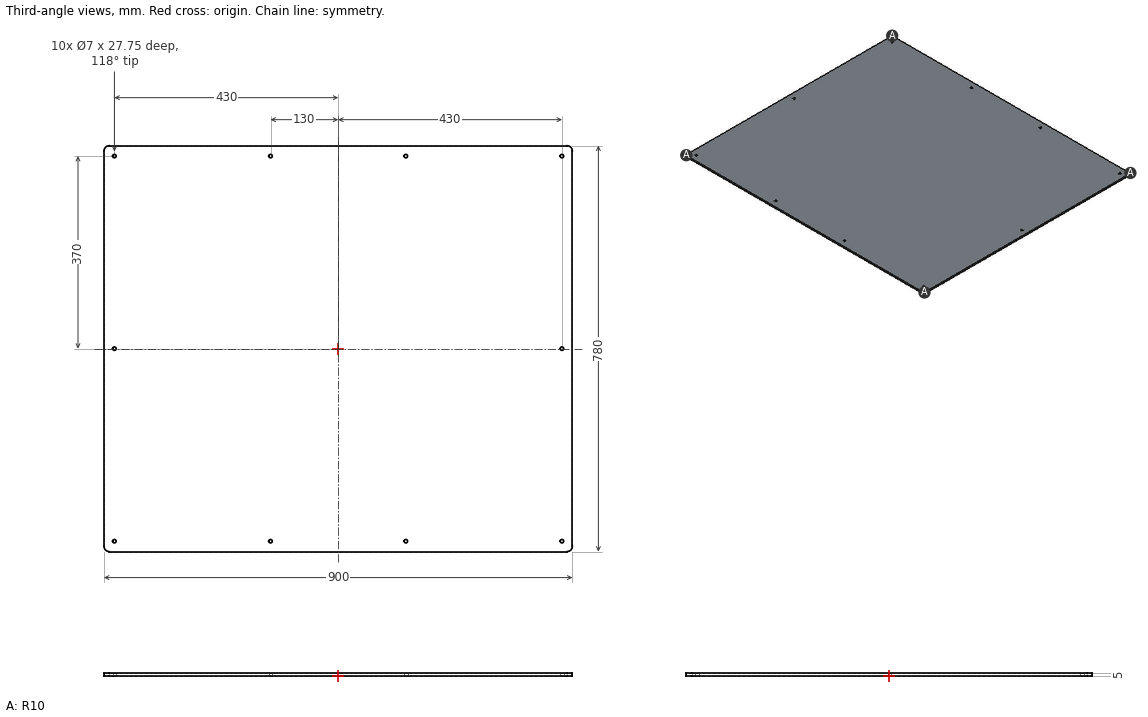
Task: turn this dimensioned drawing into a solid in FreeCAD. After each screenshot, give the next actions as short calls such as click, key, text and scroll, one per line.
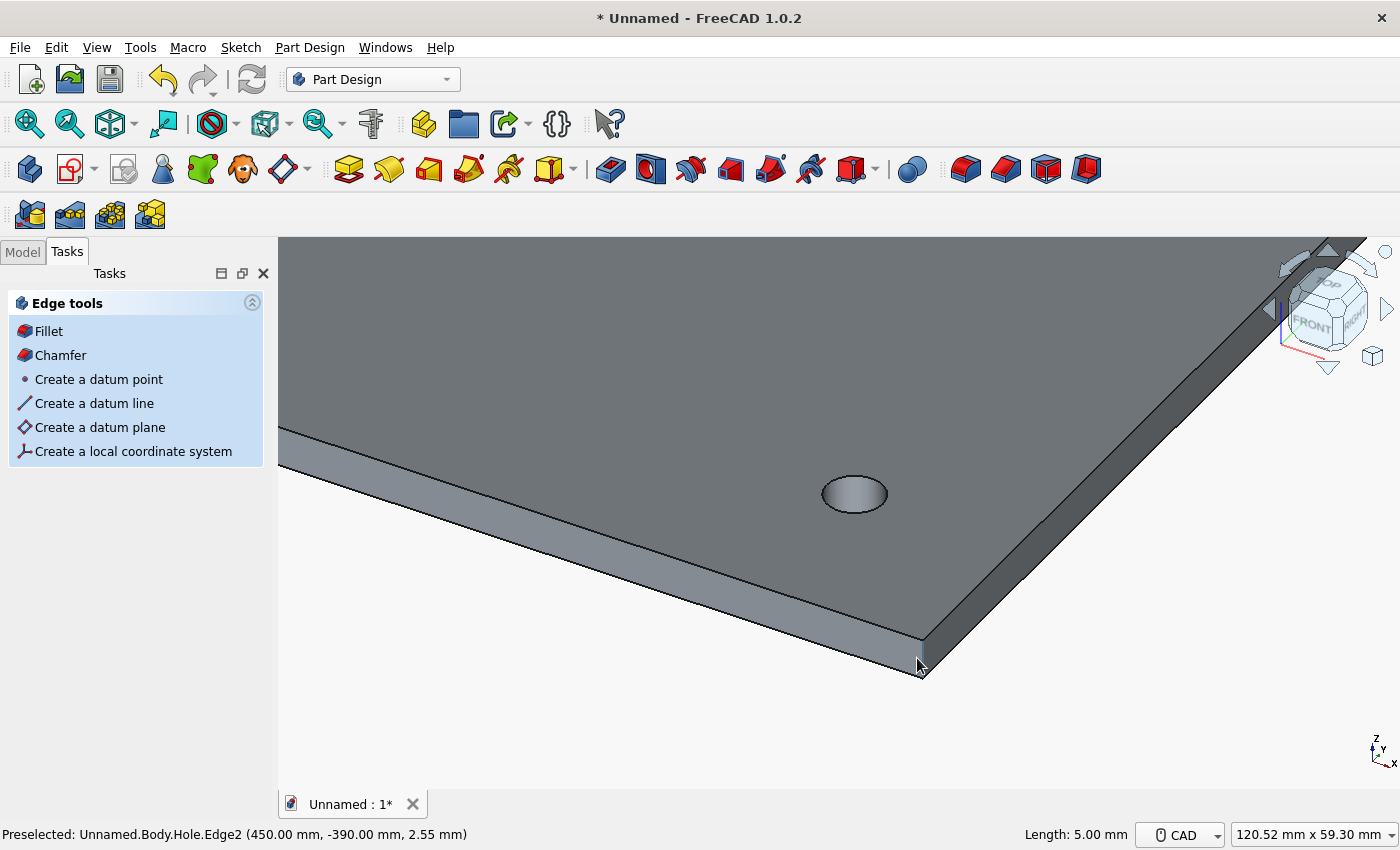
click(30, 124)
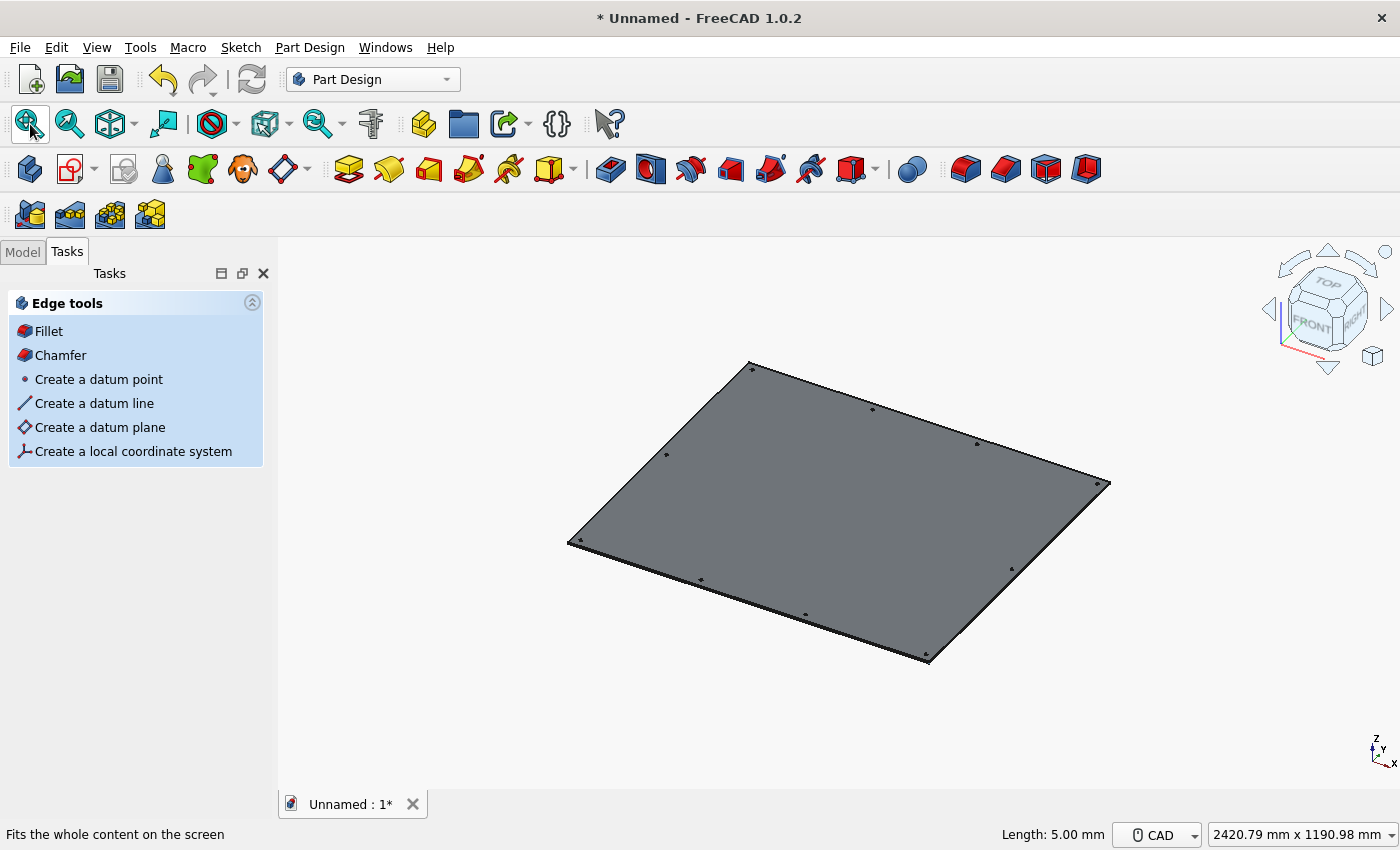
key(0)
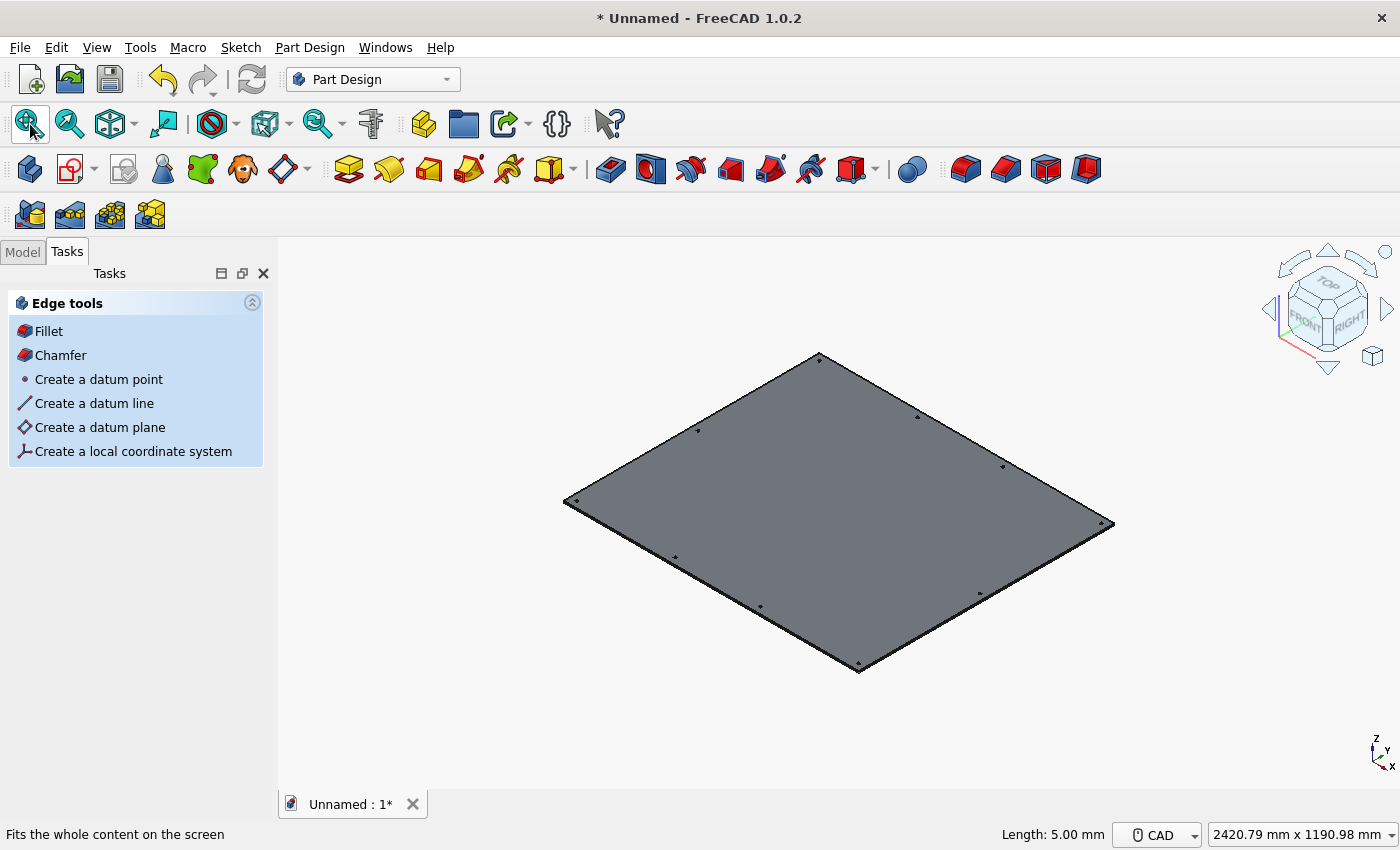
scroll(564, 501, up, 15)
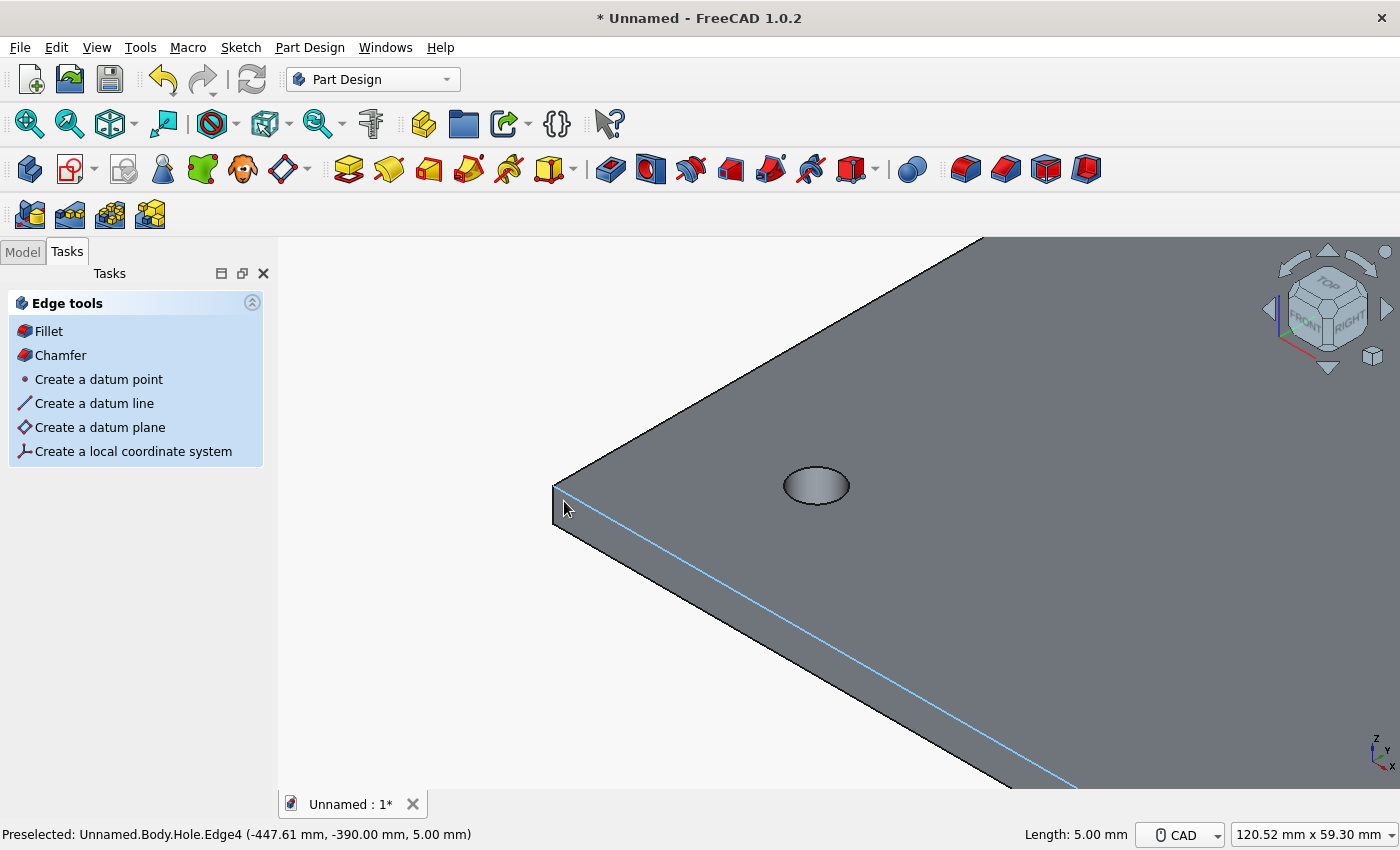
click(30, 124)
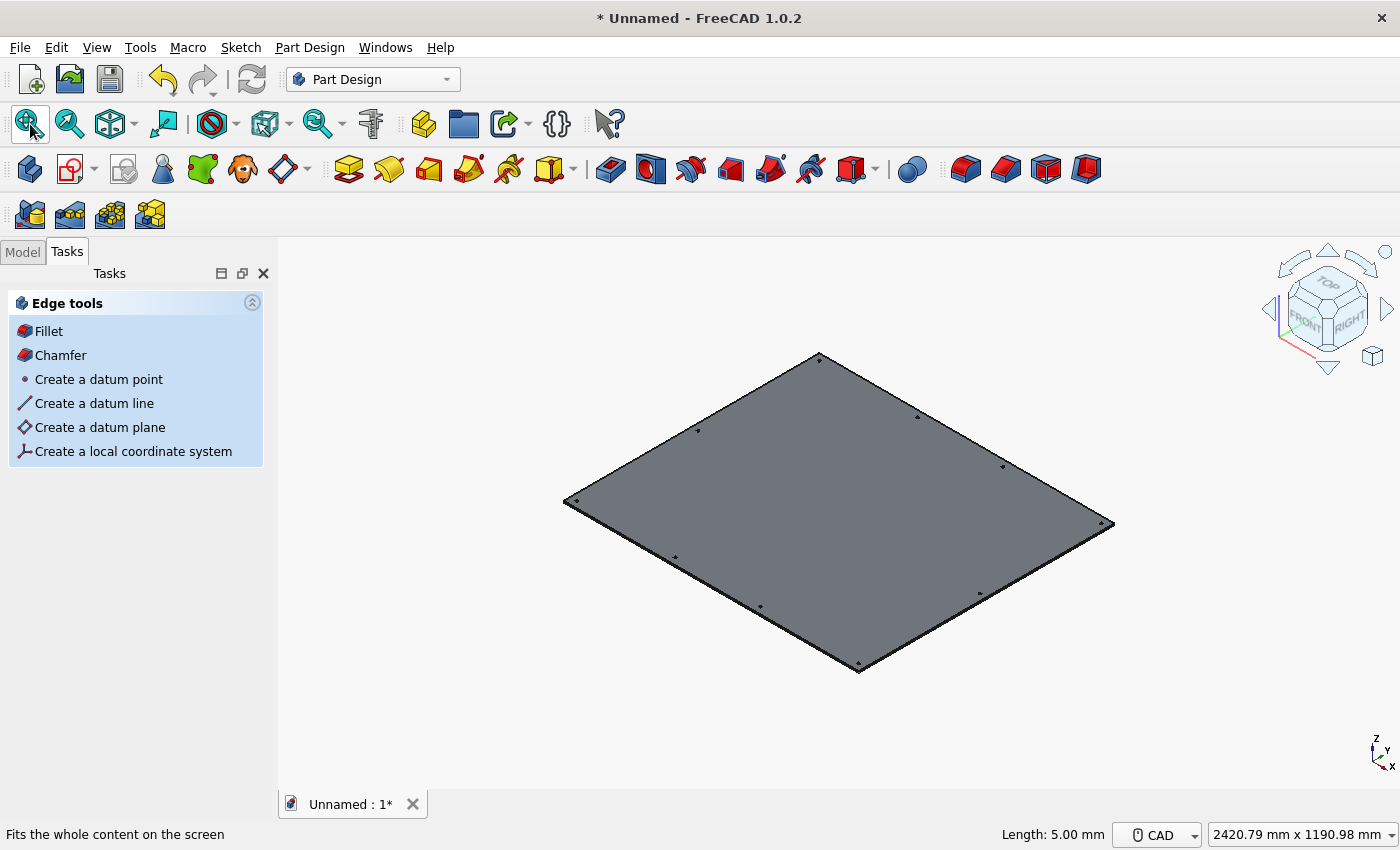
key(2)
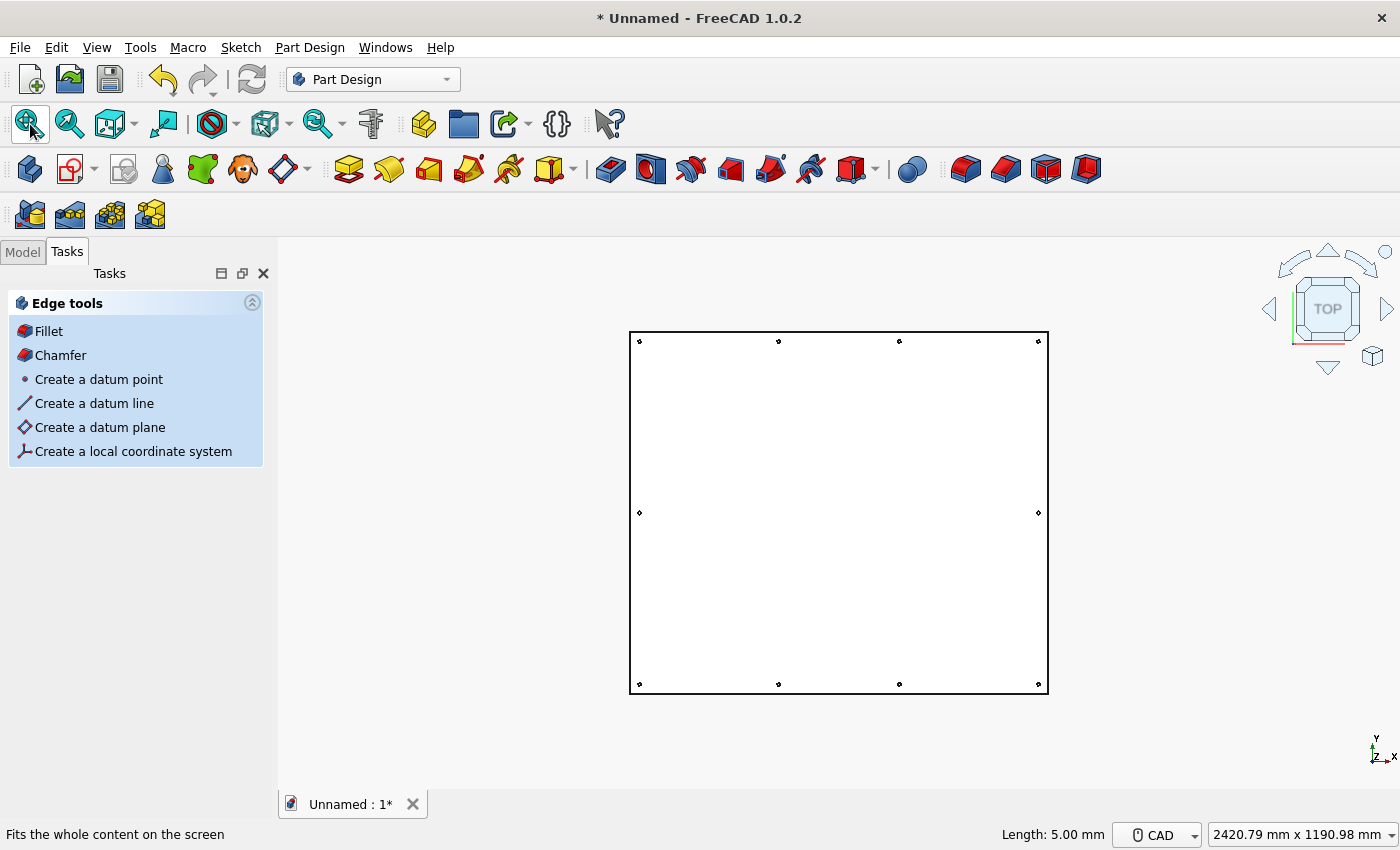
scroll(630, 693, up, 15)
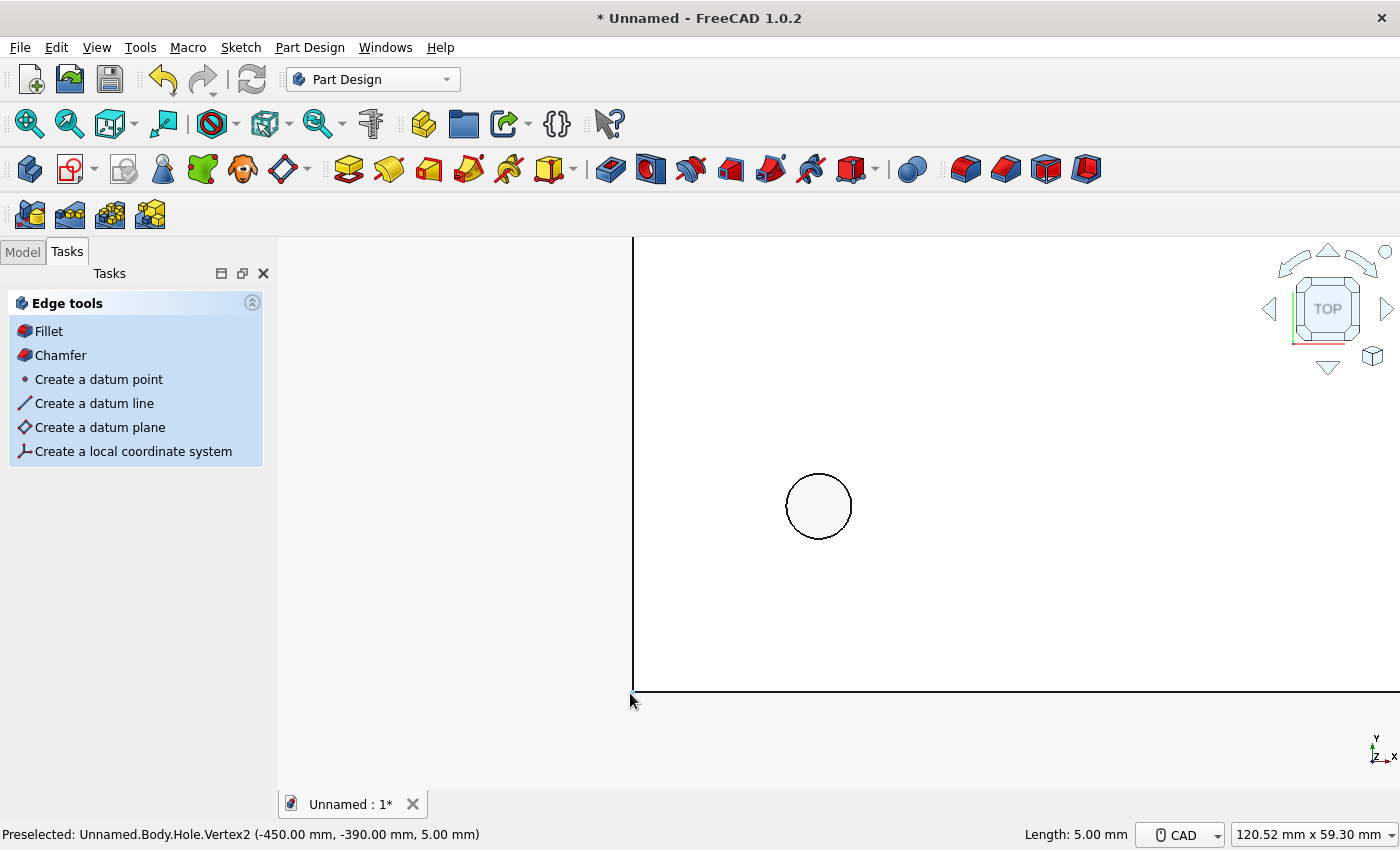
key(v)
key(f)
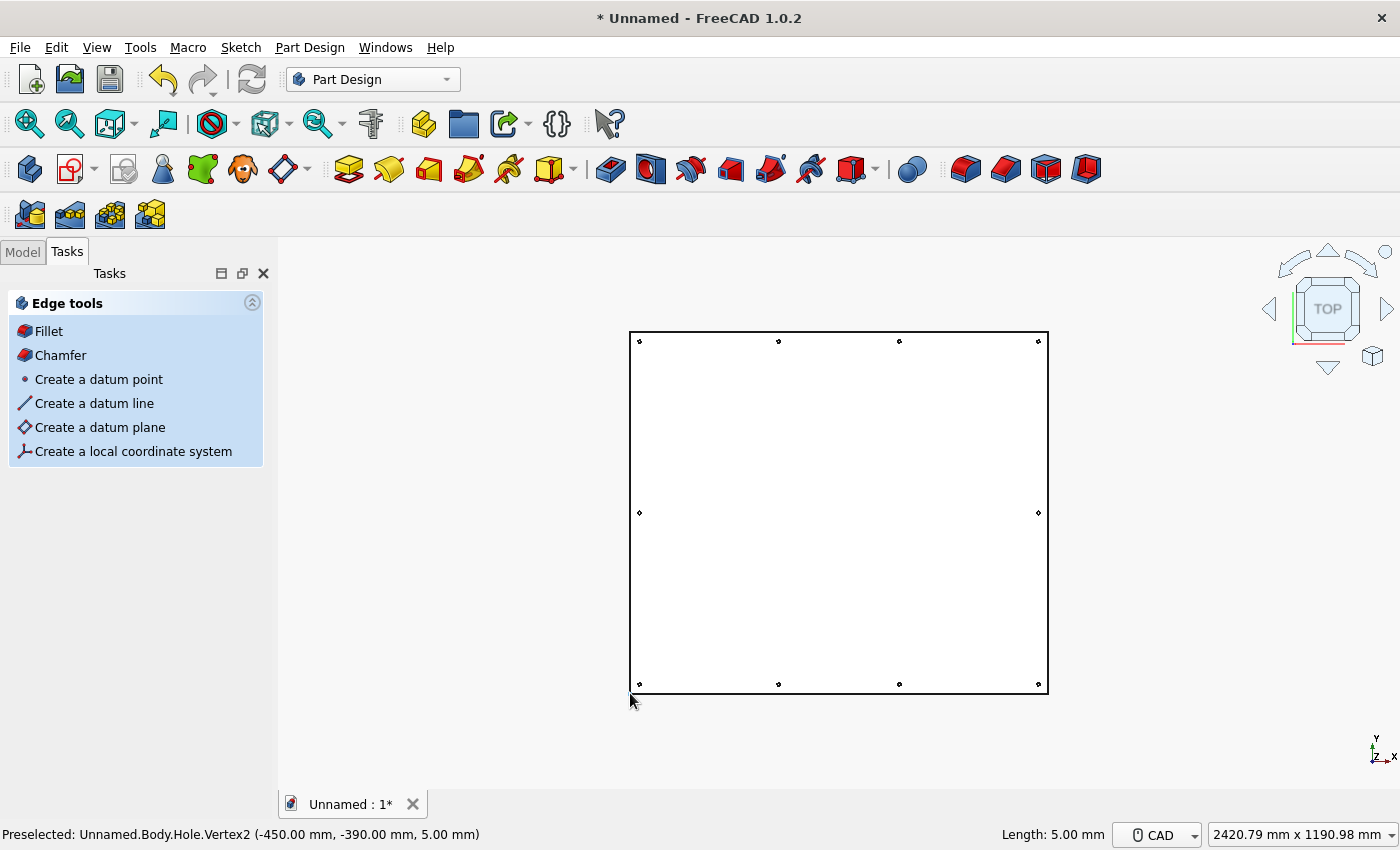
key(1)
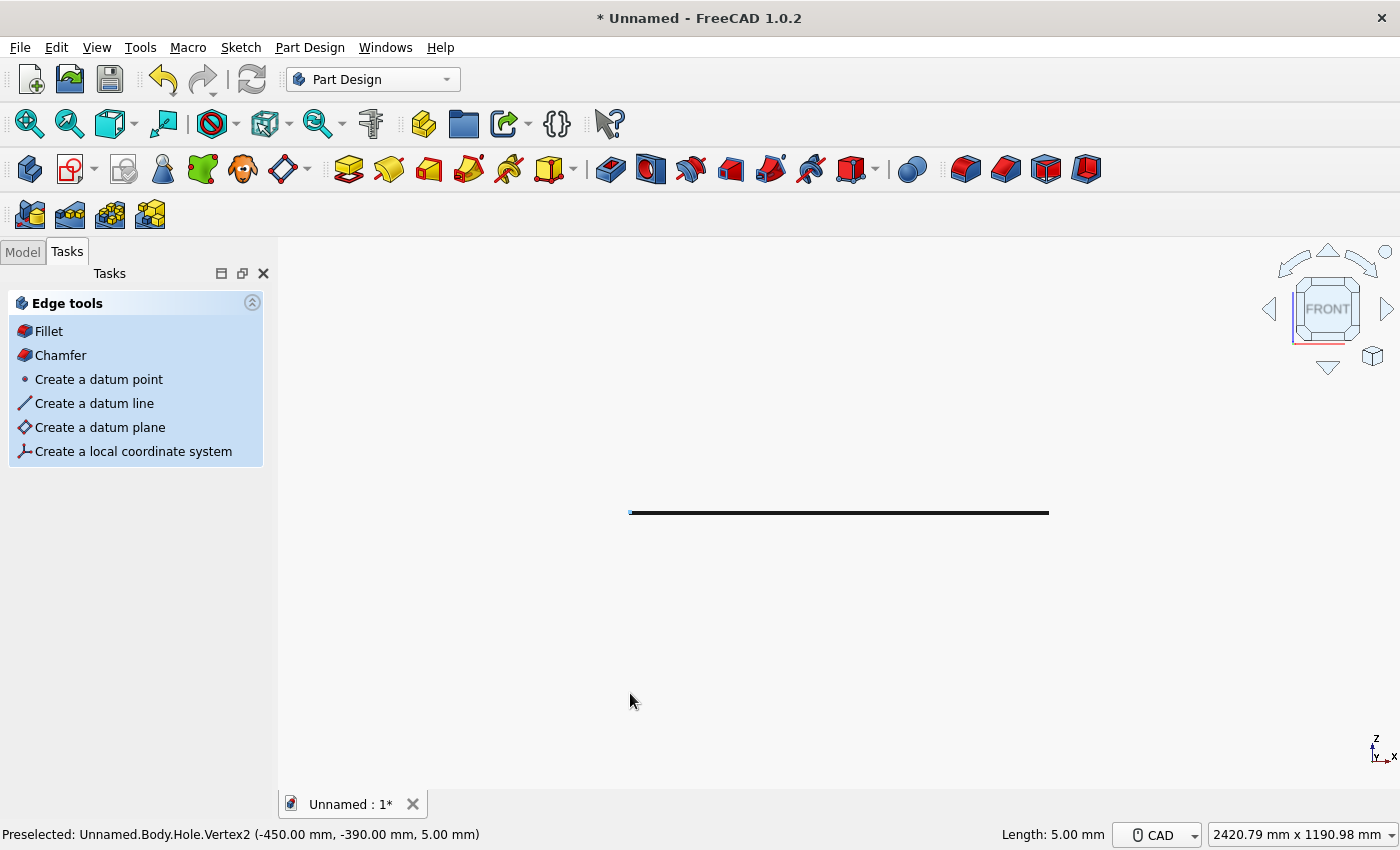
key(v)
key(f)